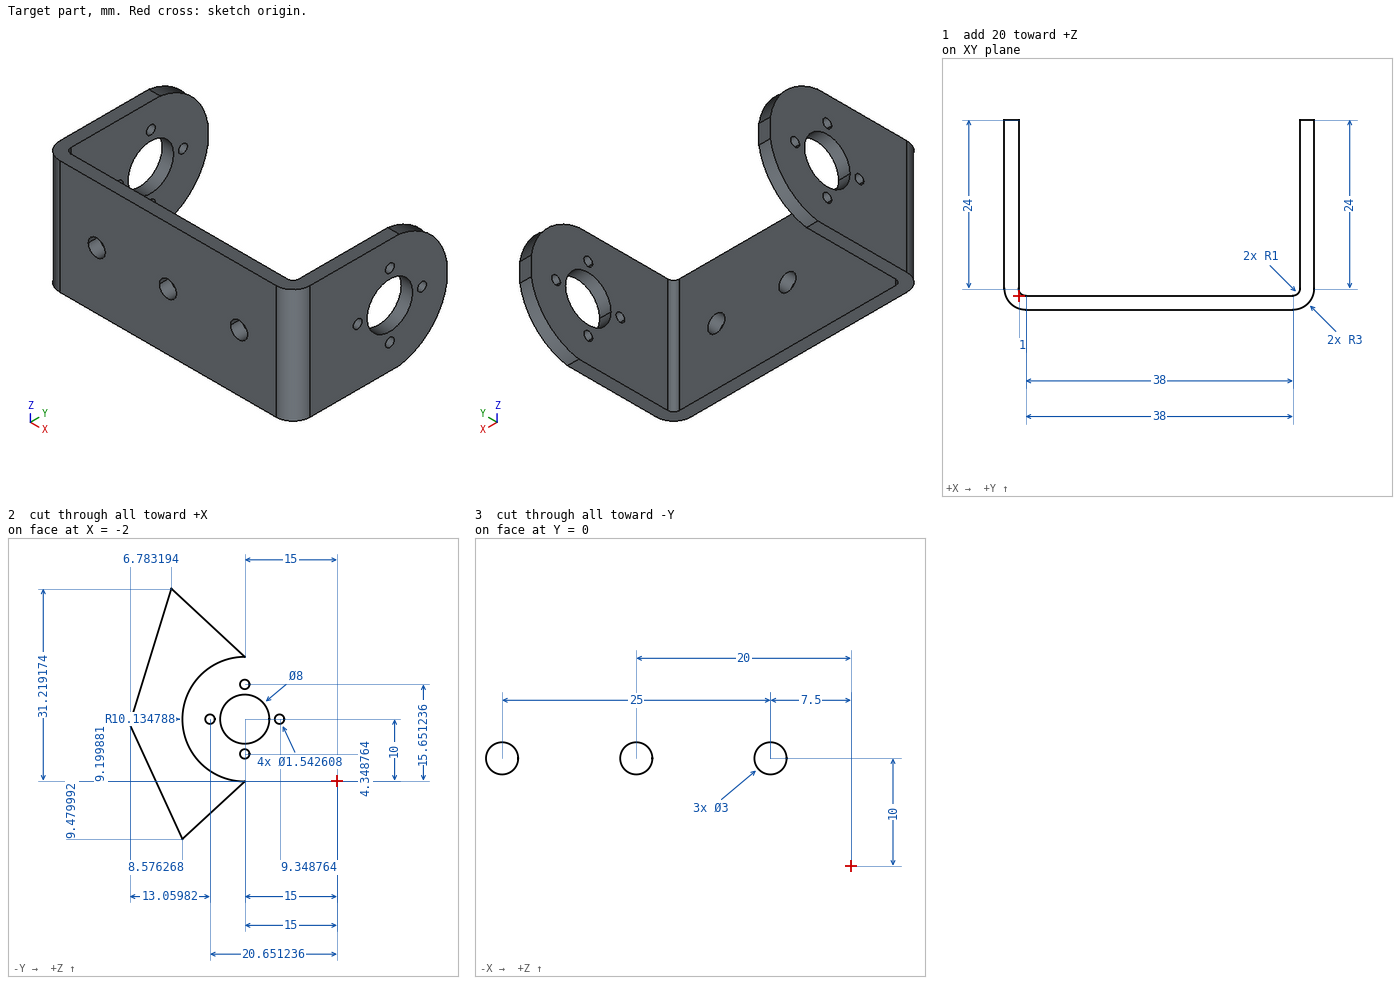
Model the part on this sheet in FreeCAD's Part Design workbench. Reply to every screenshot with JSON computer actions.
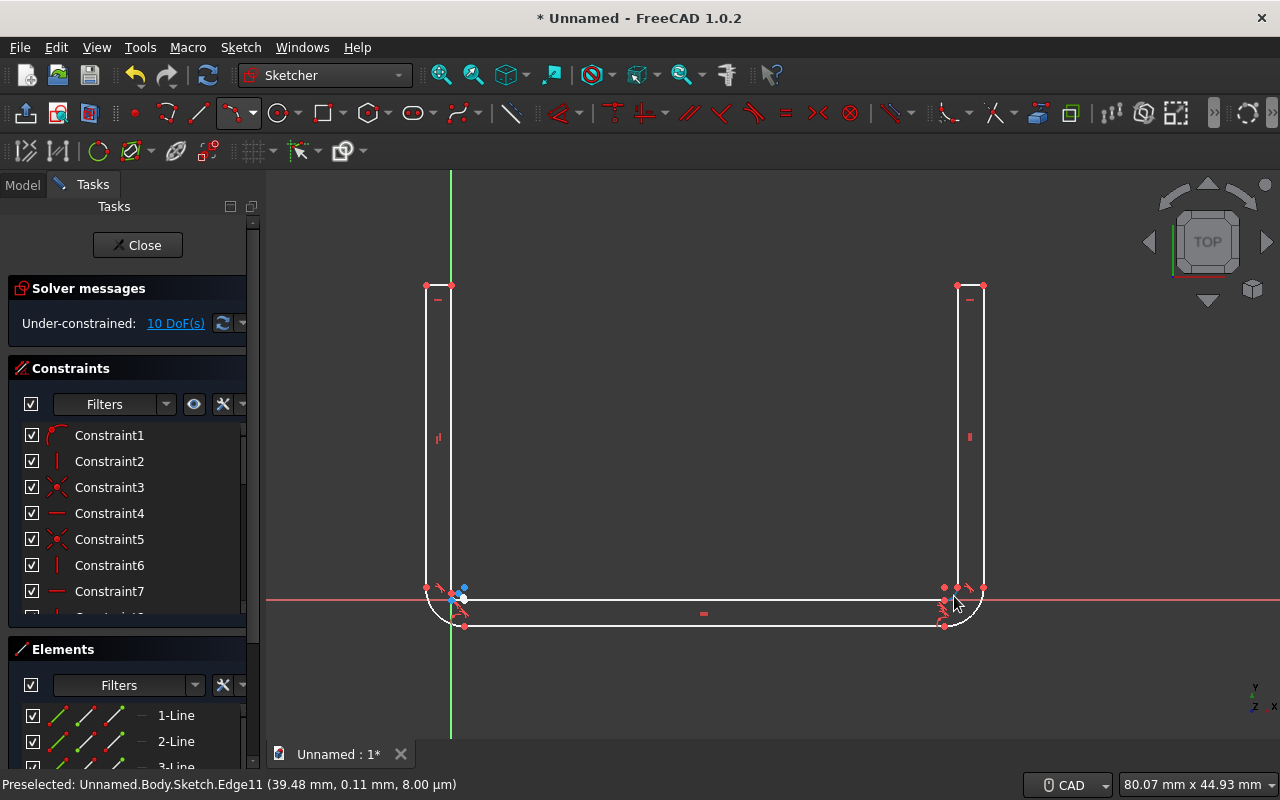
{"action": "left_click", "coordinate": [437, 615]}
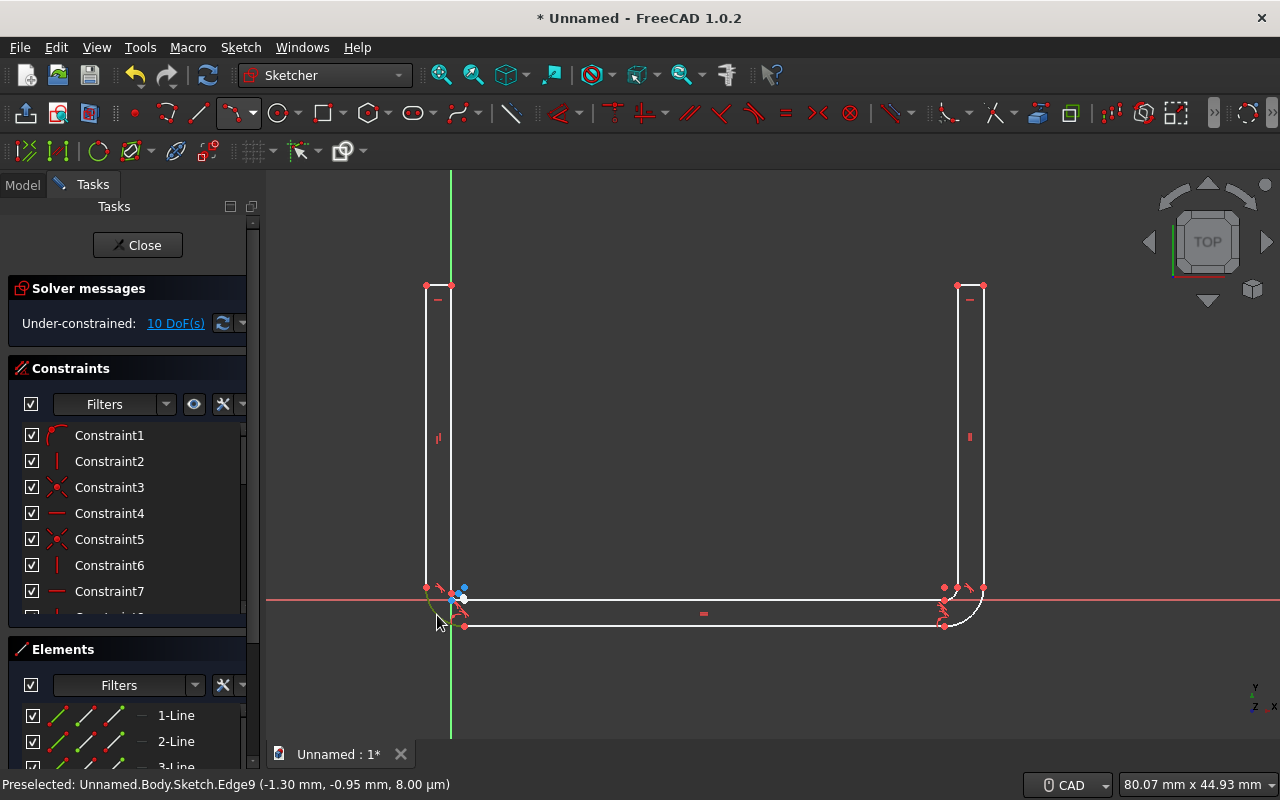
{"action": "scroll", "coordinate": [453, 598], "scroll_direction": "up", "scroll_amount": 6}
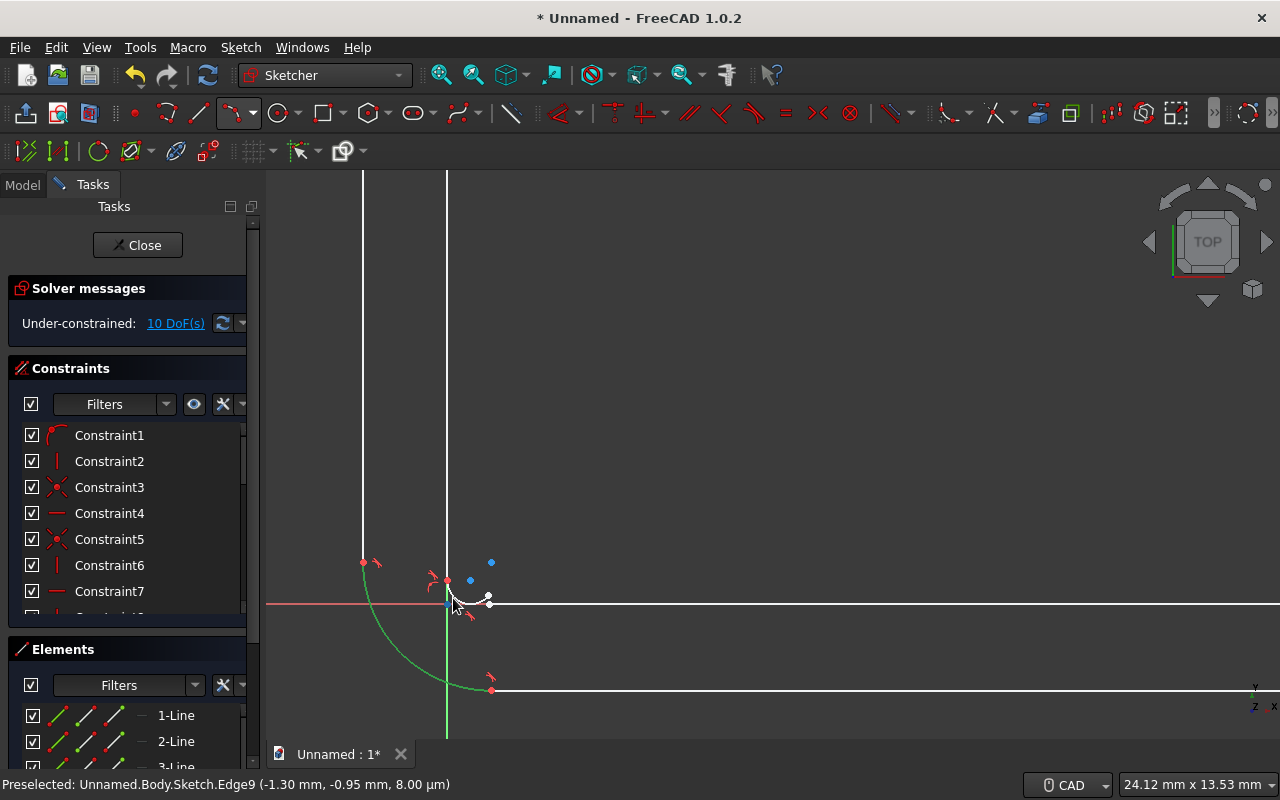
{"action": "left_click", "coordinate": [454, 597]}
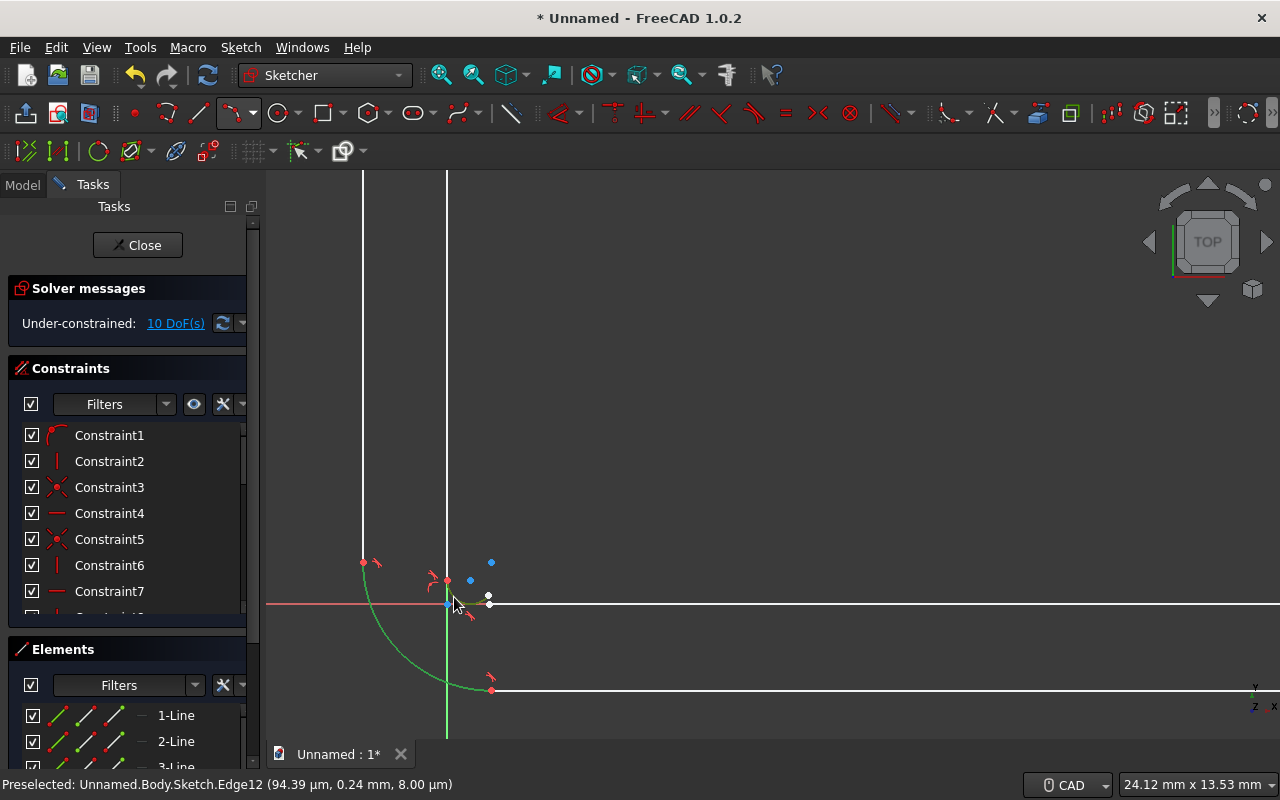
{"action": "left_click", "coordinate": [614, 114]}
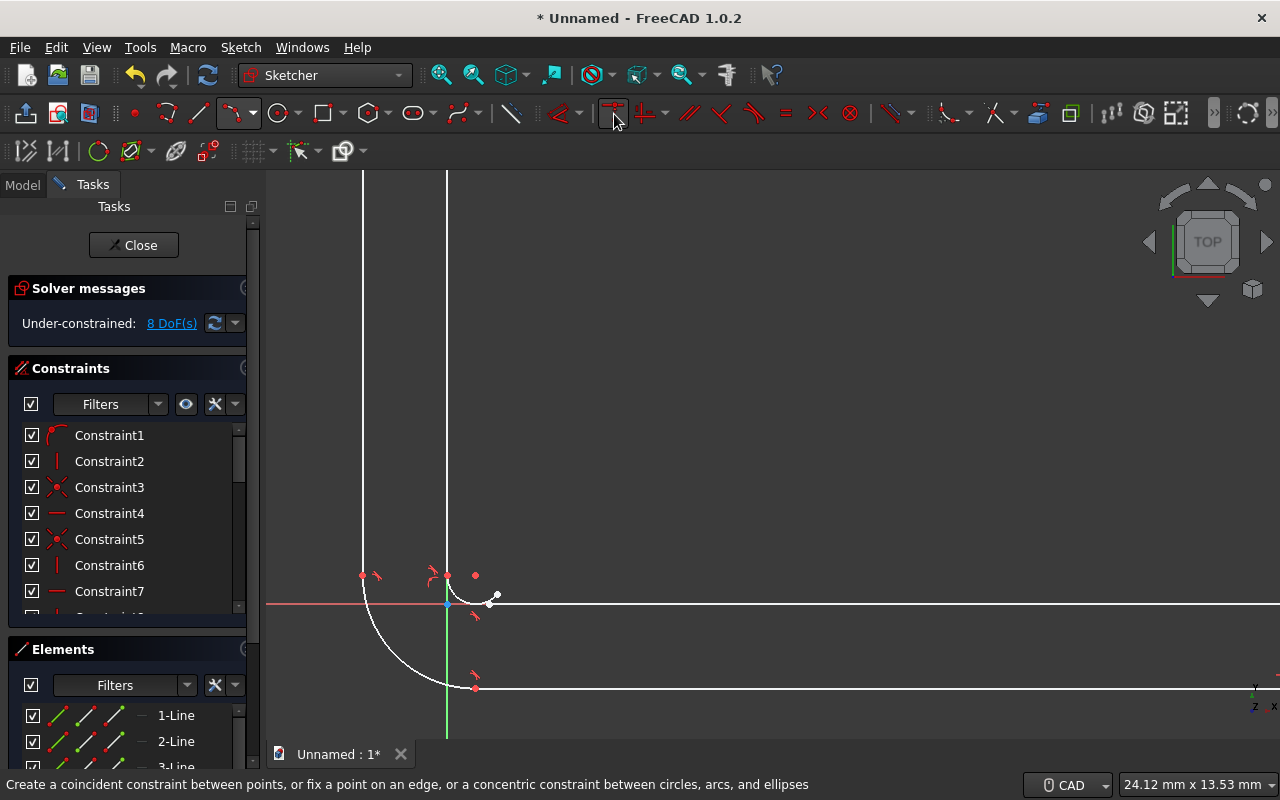
{"action": "left_click", "coordinate": [375, 627]}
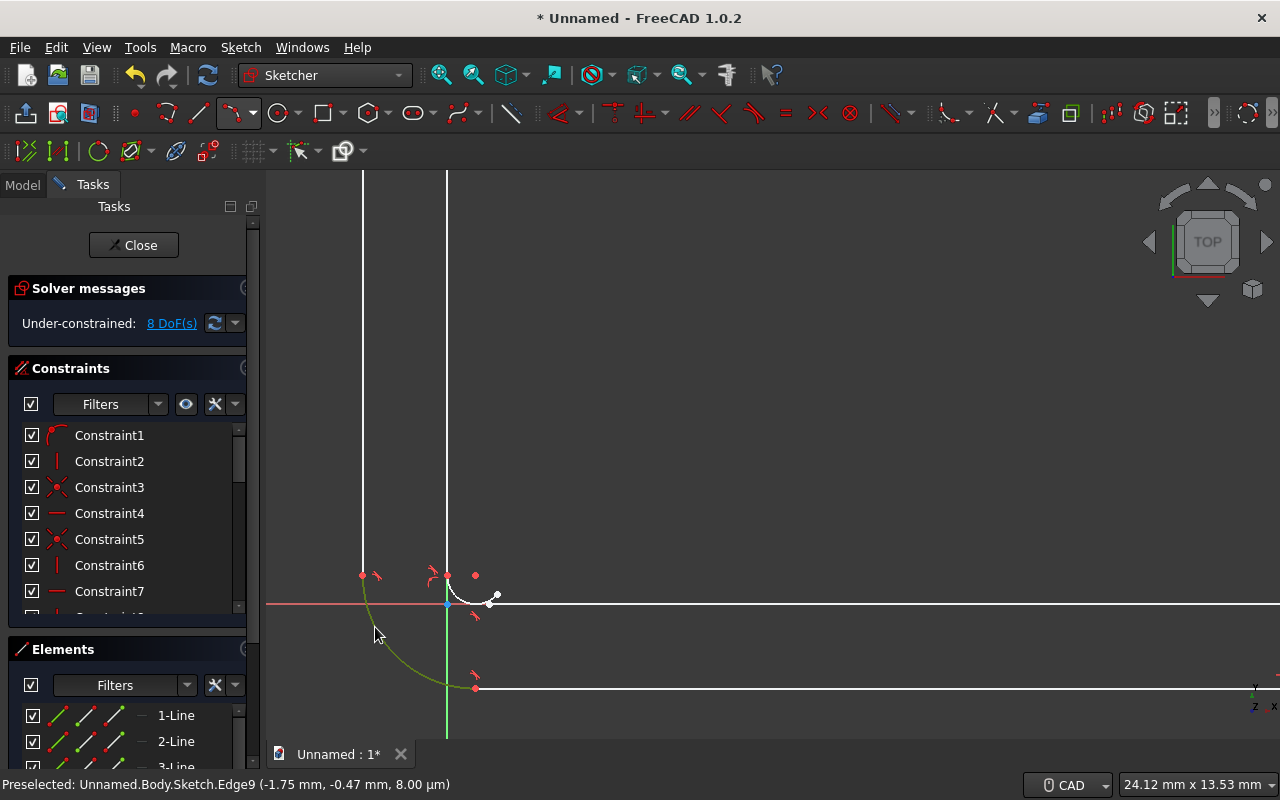
{"action": "scroll", "coordinate": [453, 598], "scroll_direction": "down", "scroll_amount": 6}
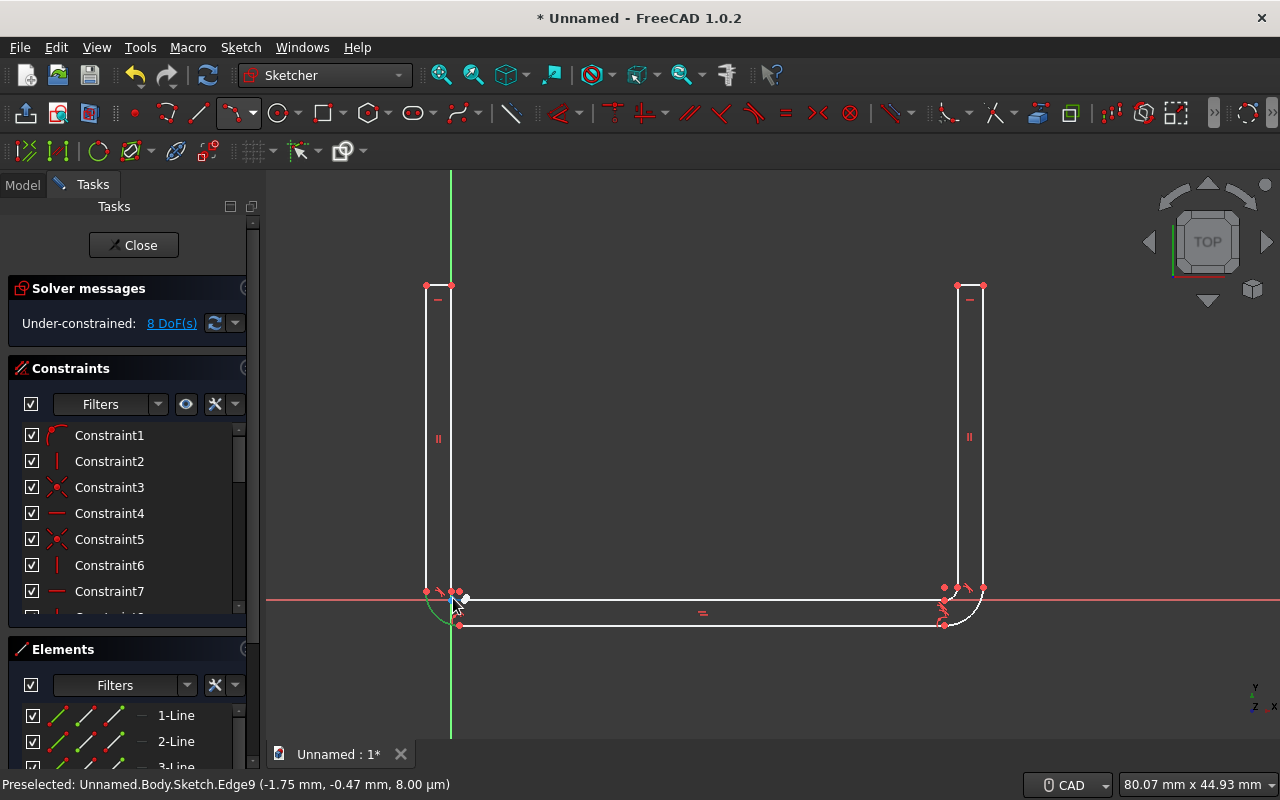
{"action": "left_click", "coordinate": [962, 622]}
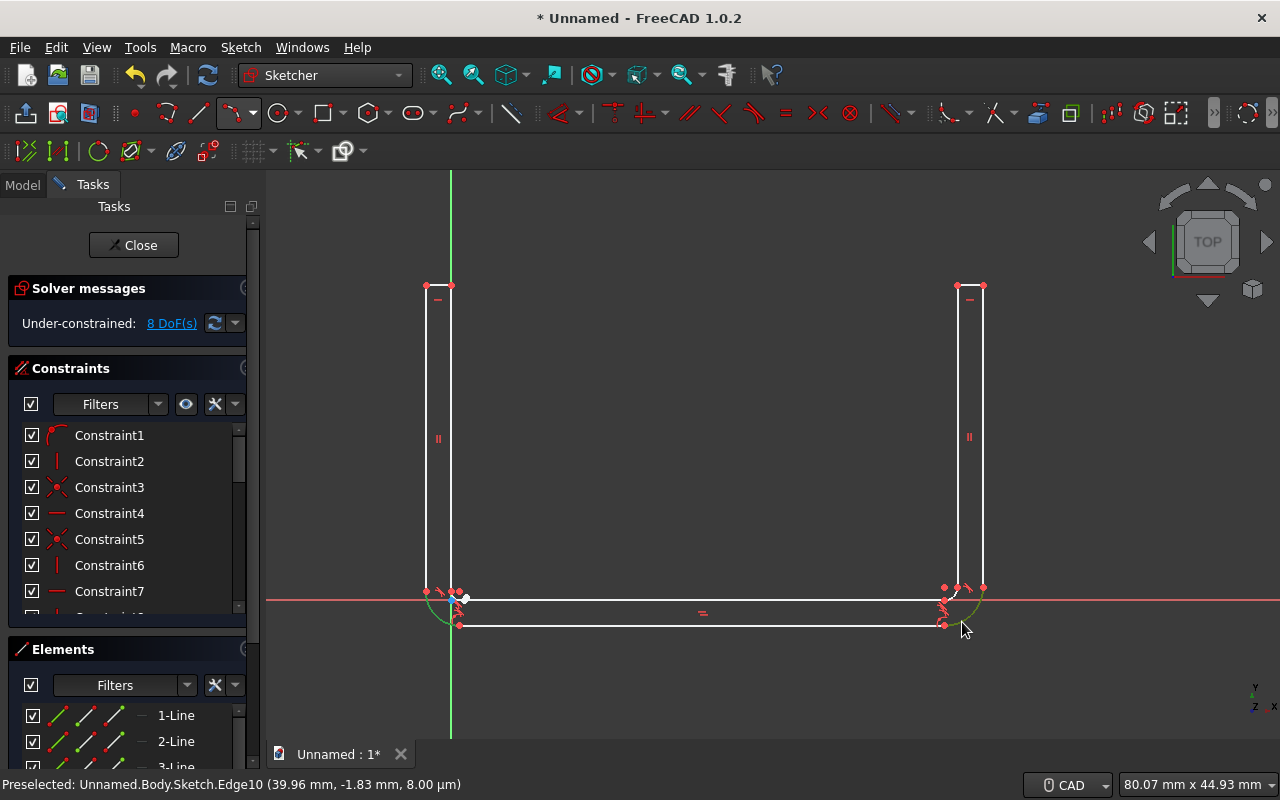
{"action": "left_click", "coordinate": [786, 114]}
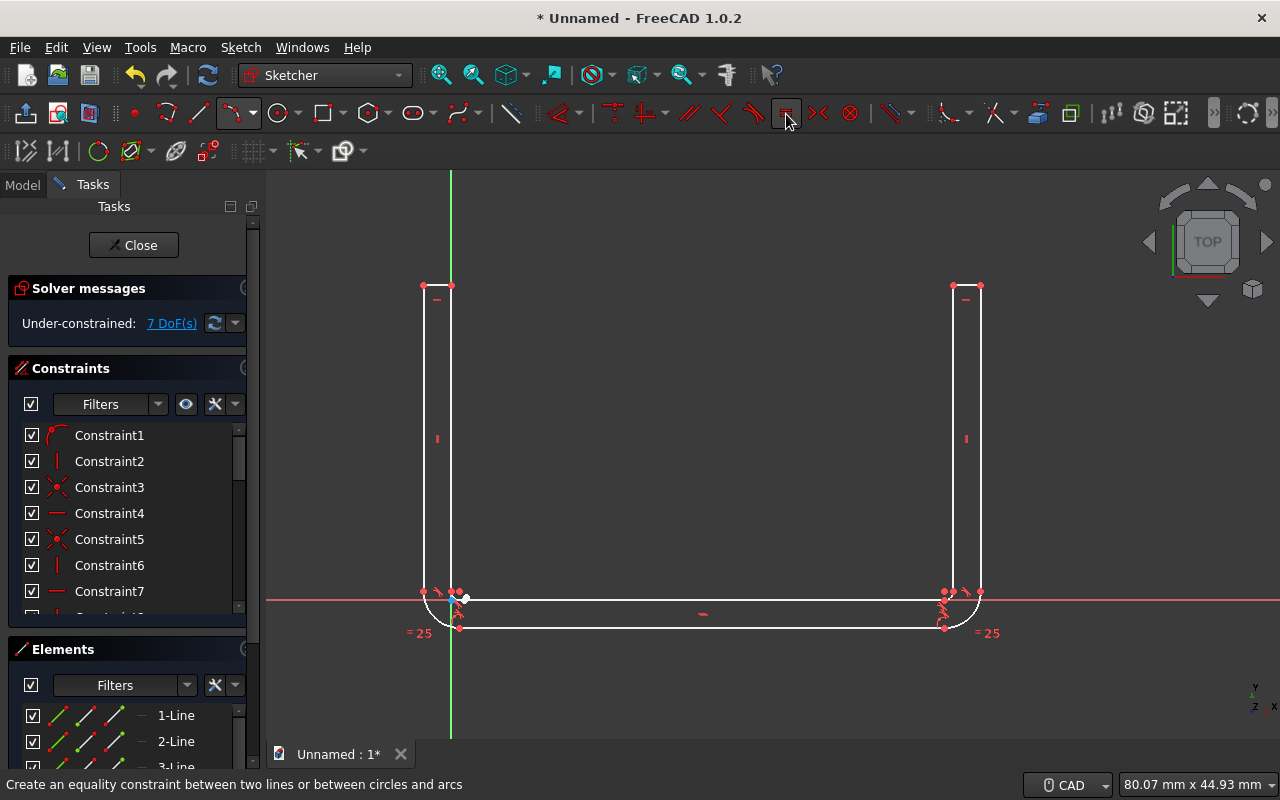
{"action": "left_click", "coordinate": [558, 114]}